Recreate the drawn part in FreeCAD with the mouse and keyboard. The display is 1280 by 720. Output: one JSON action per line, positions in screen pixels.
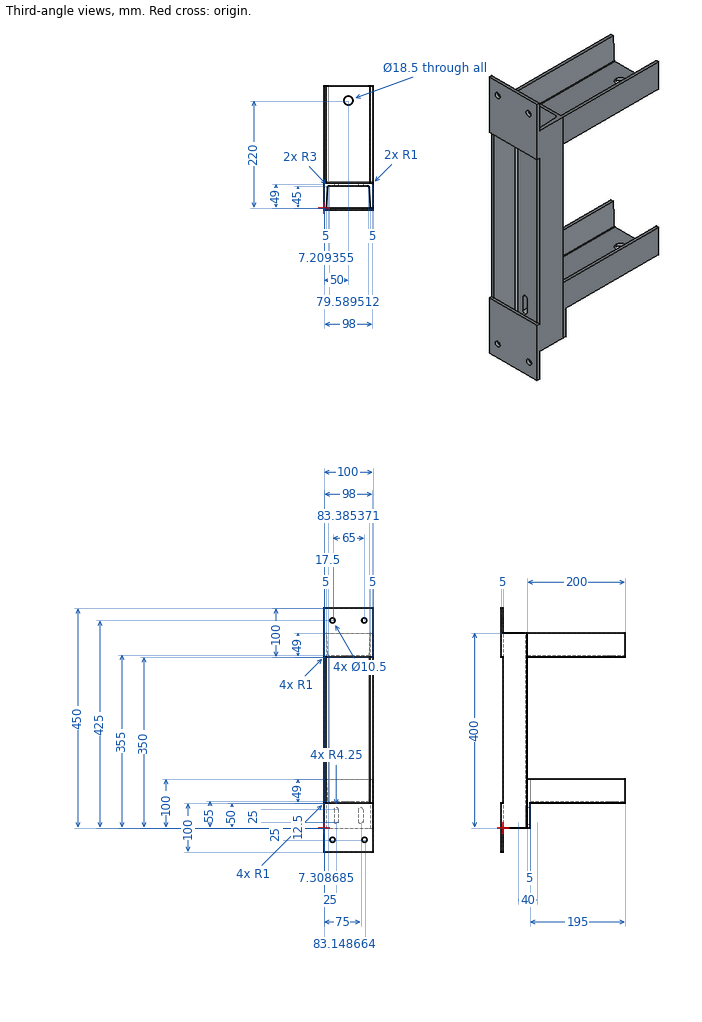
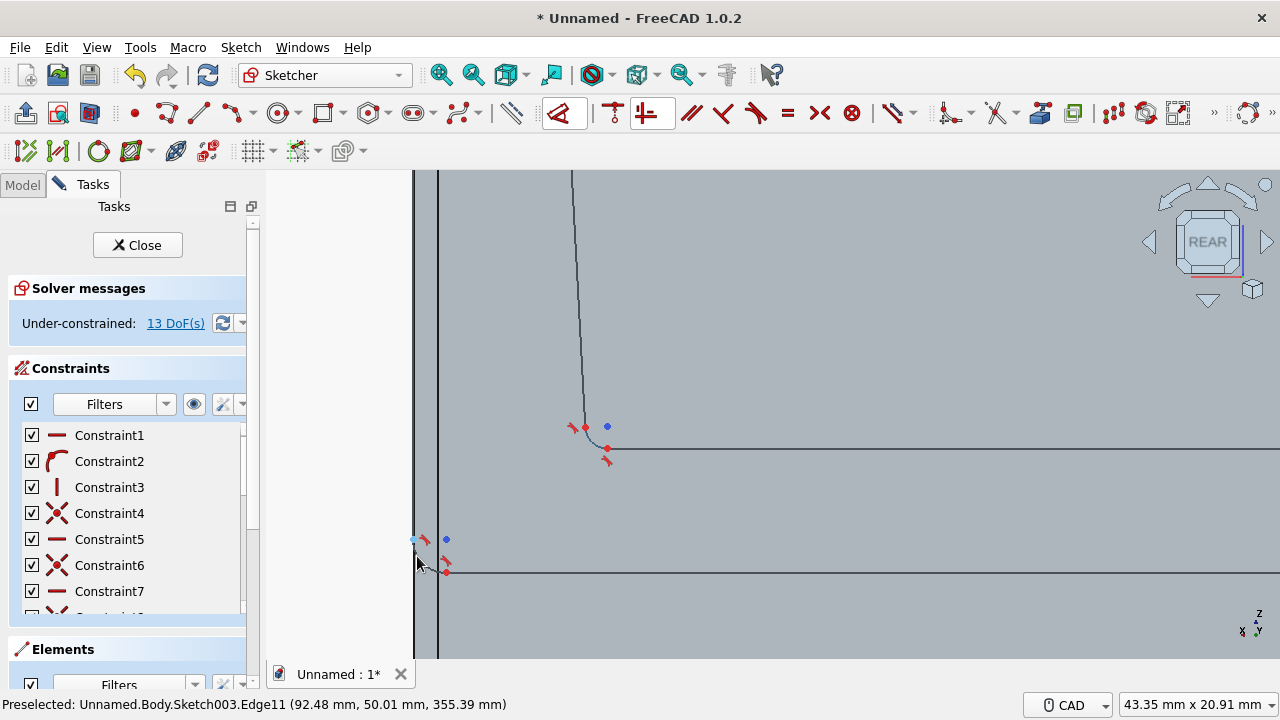
{"action": "left_click", "coordinate": [417, 555]}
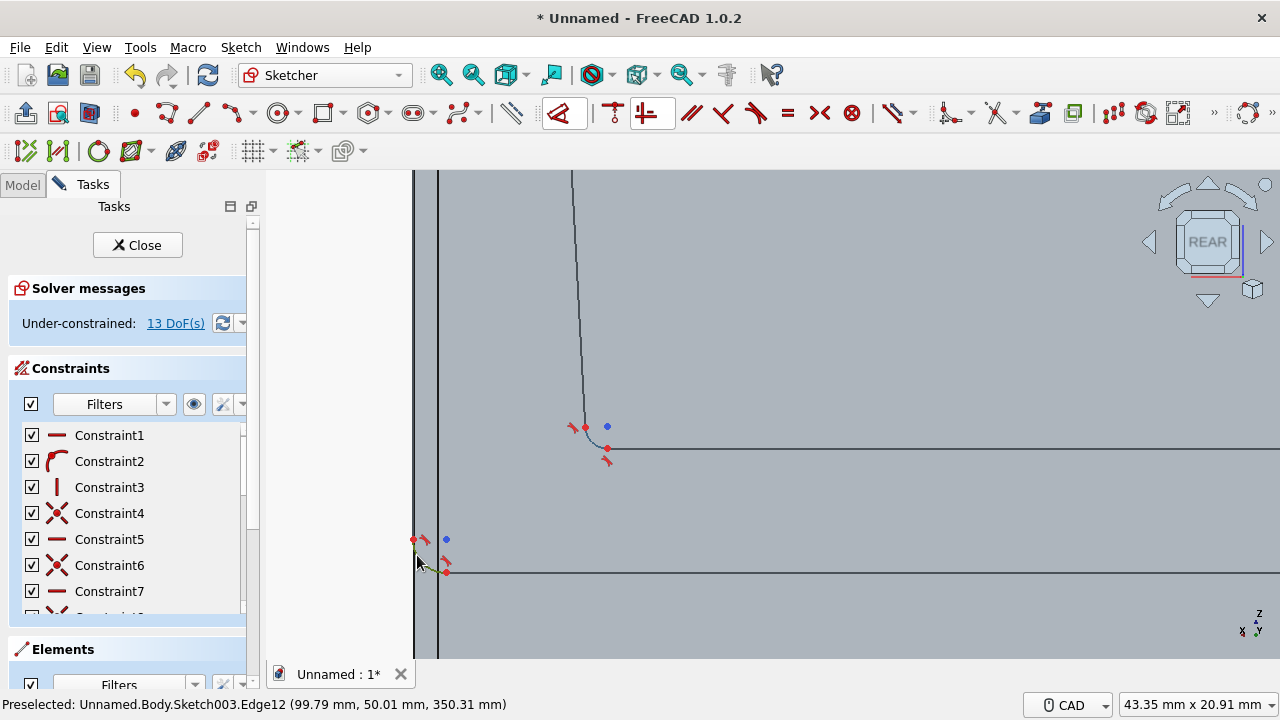
{"action": "left_click", "coordinate": [788, 114]}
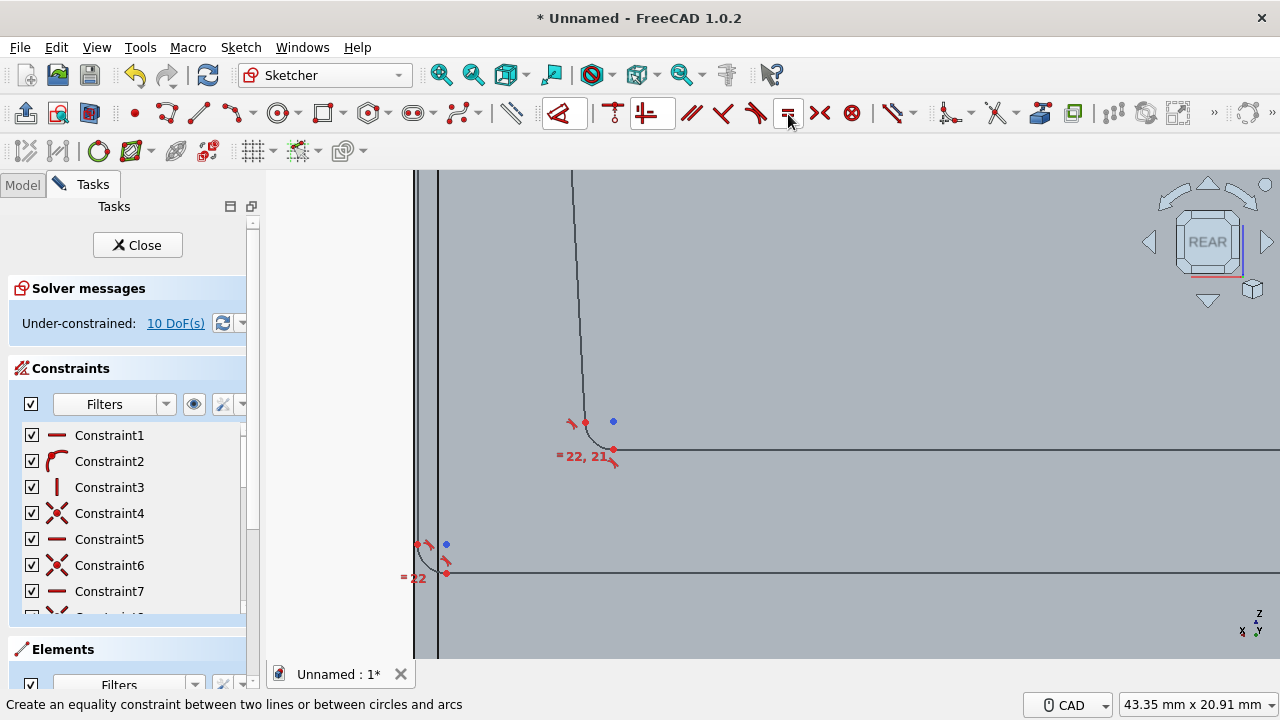
{"action": "scroll", "coordinate": [417, 556], "scroll_direction": "down", "scroll_amount": 7}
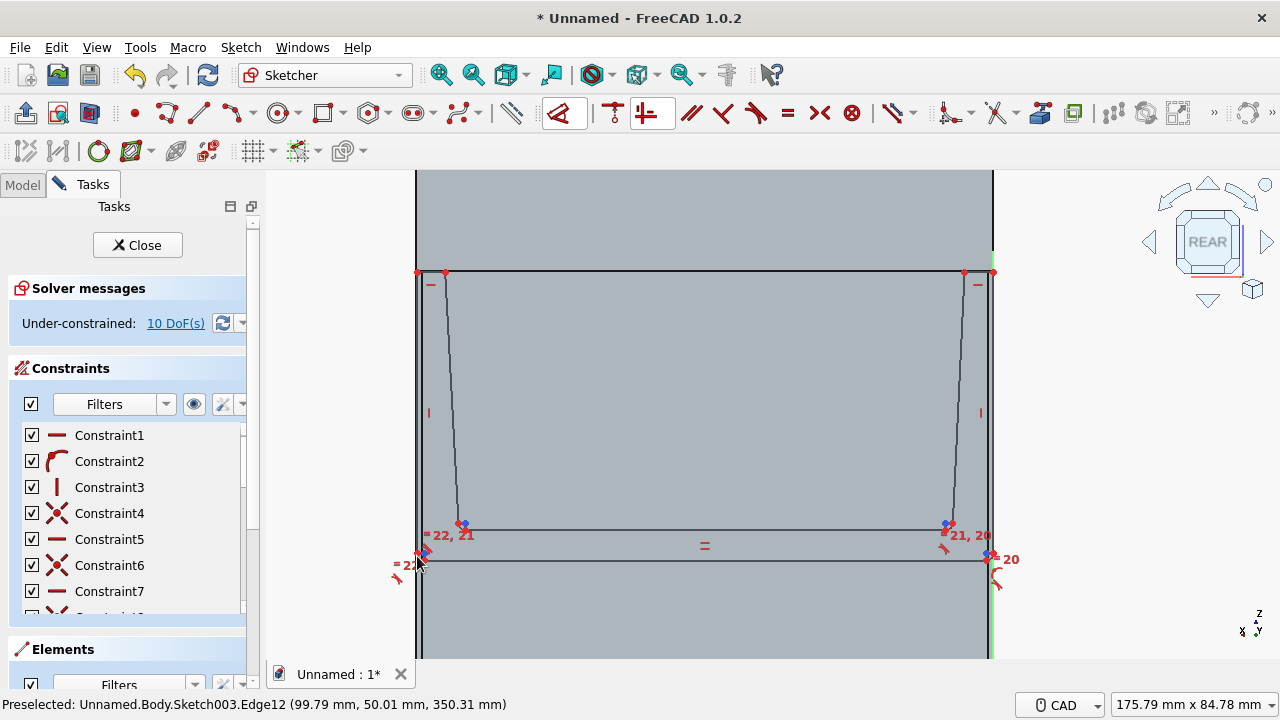
{"action": "scroll", "coordinate": [989, 560], "scroll_direction": "up", "scroll_amount": 10}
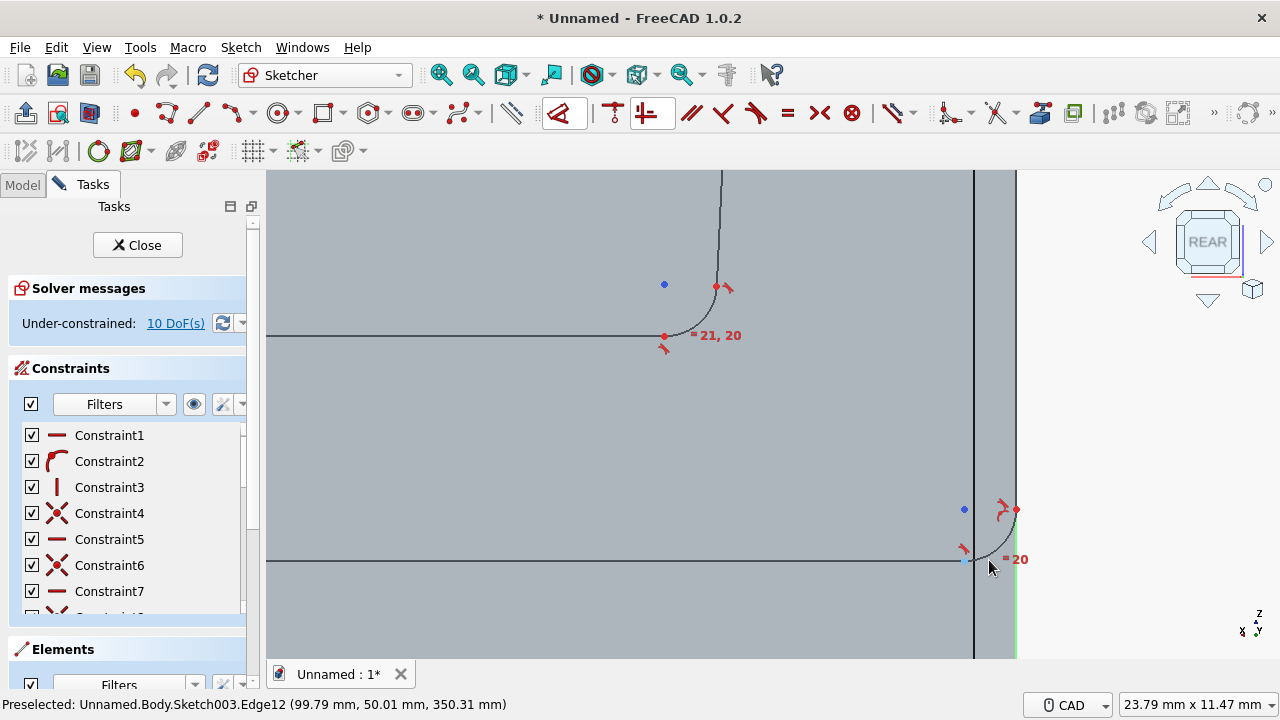
{"action": "left_click", "coordinate": [988, 555]}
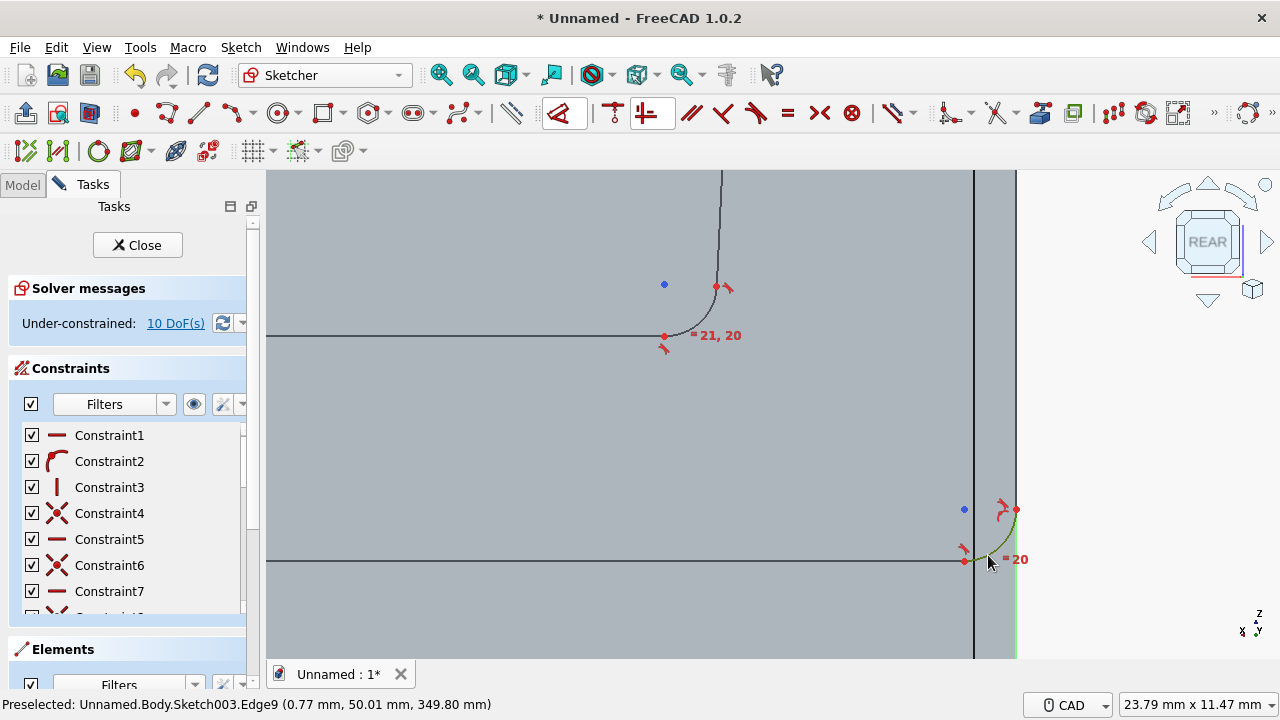
{"action": "key", "text": "k r"}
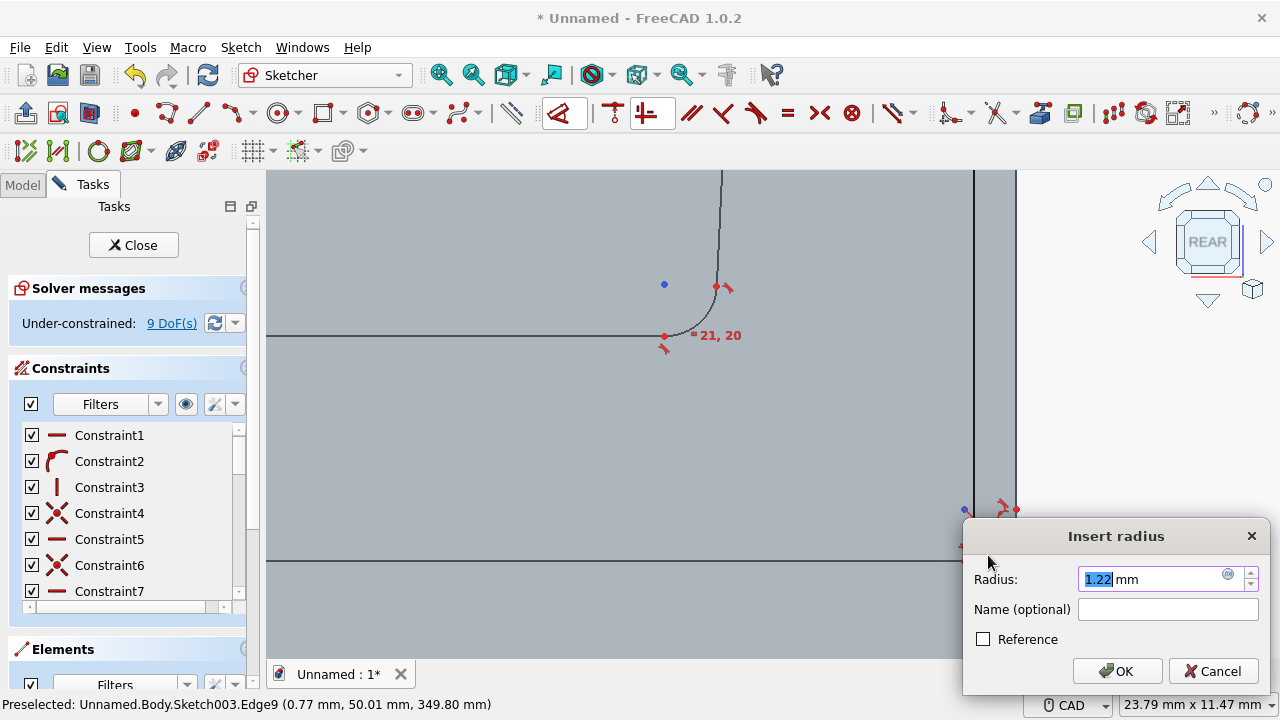
{"action": "type", "text": "1"}
{"action": "key", "text": "Return"}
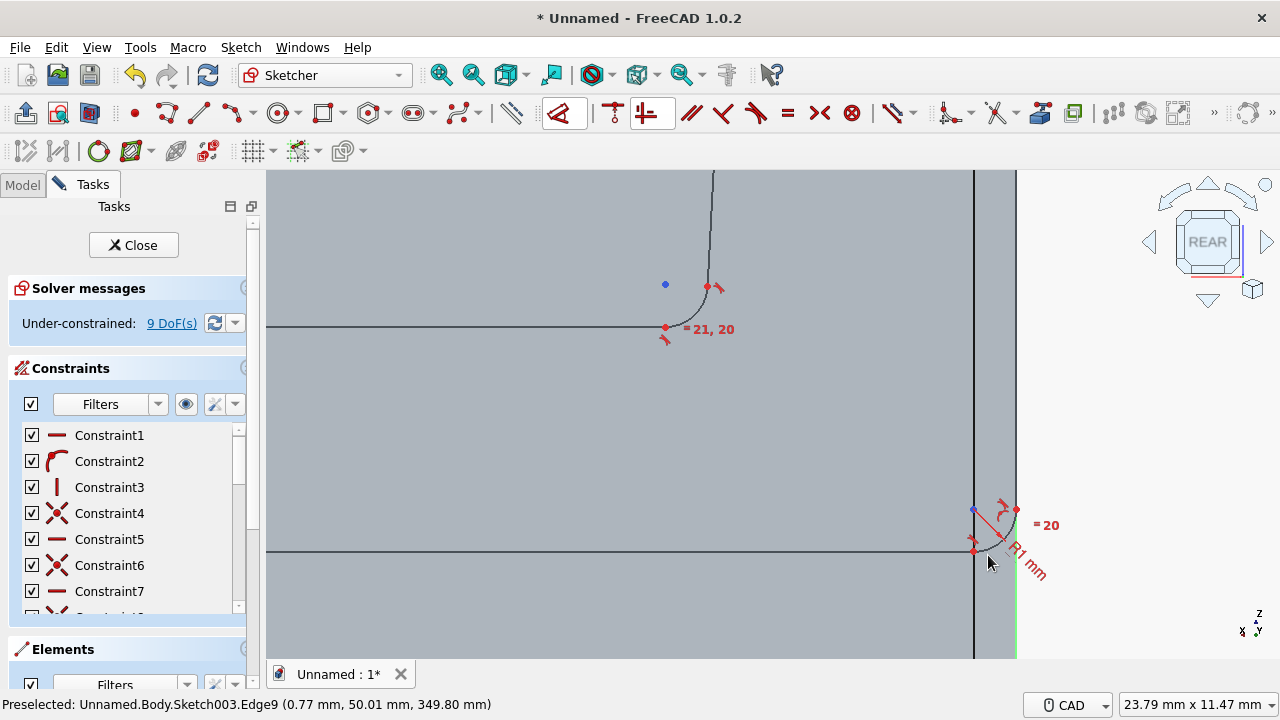
{"action": "scroll", "coordinate": [989, 560], "scroll_direction": "down", "scroll_amount": 10}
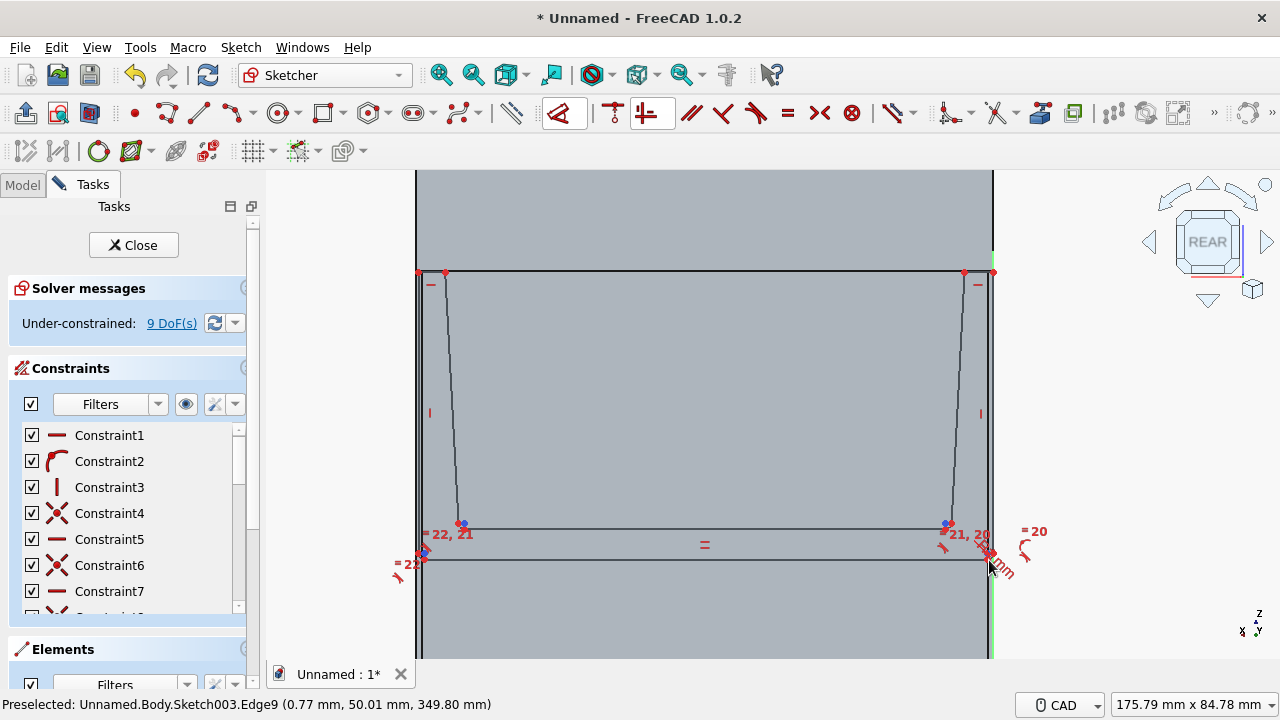
{"action": "scroll", "coordinate": [985, 272], "scroll_direction": "up", "scroll_amount": 3}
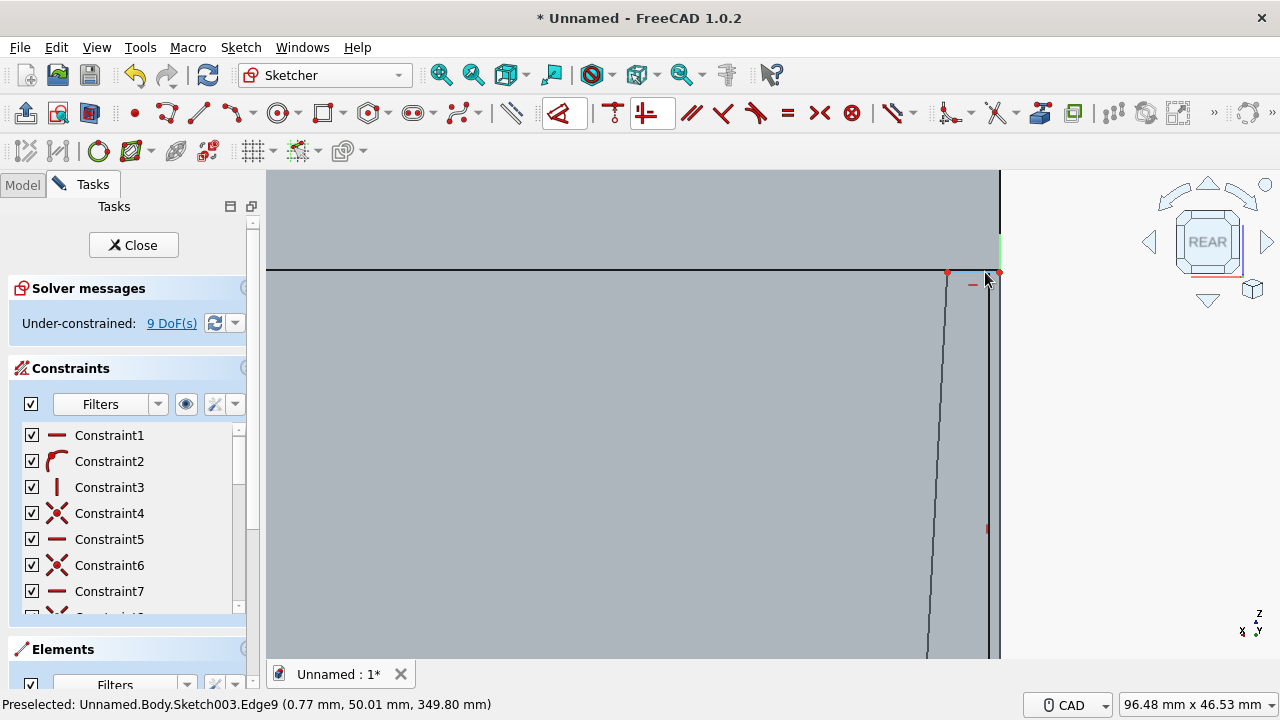
{"action": "left_click", "coordinate": [984, 272]}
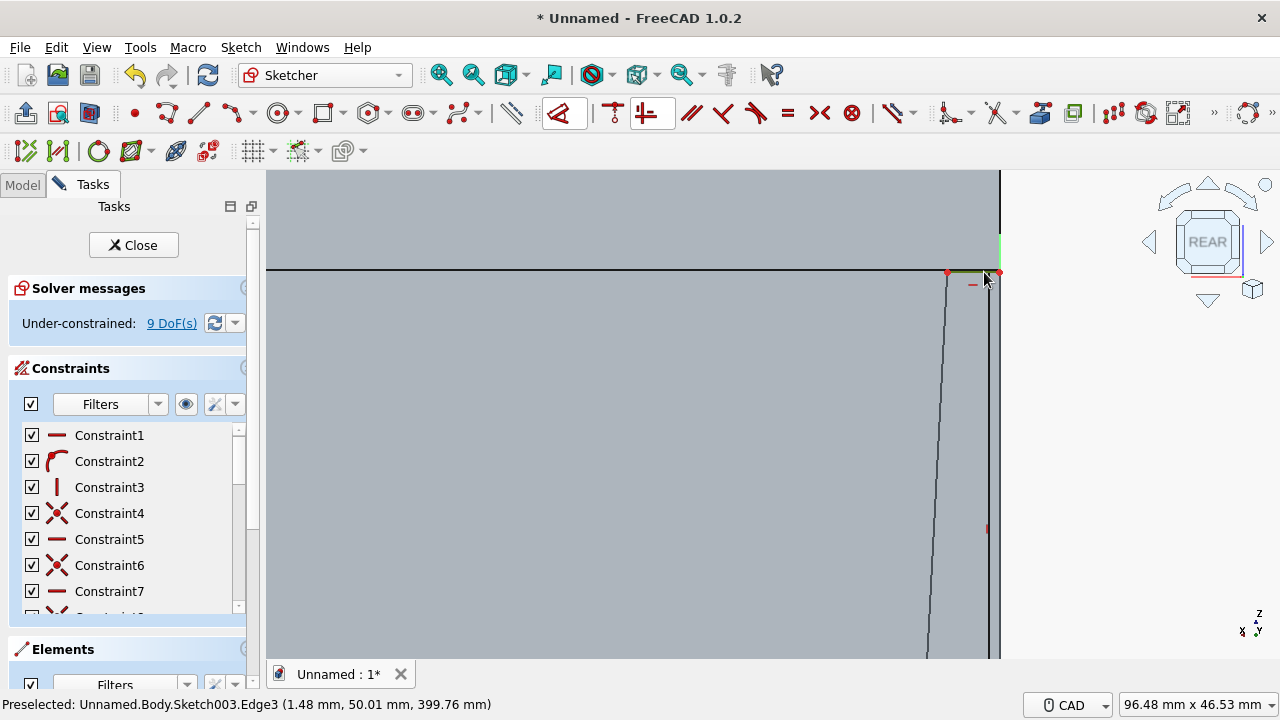
{"action": "left_click", "coordinate": [582, 114]}